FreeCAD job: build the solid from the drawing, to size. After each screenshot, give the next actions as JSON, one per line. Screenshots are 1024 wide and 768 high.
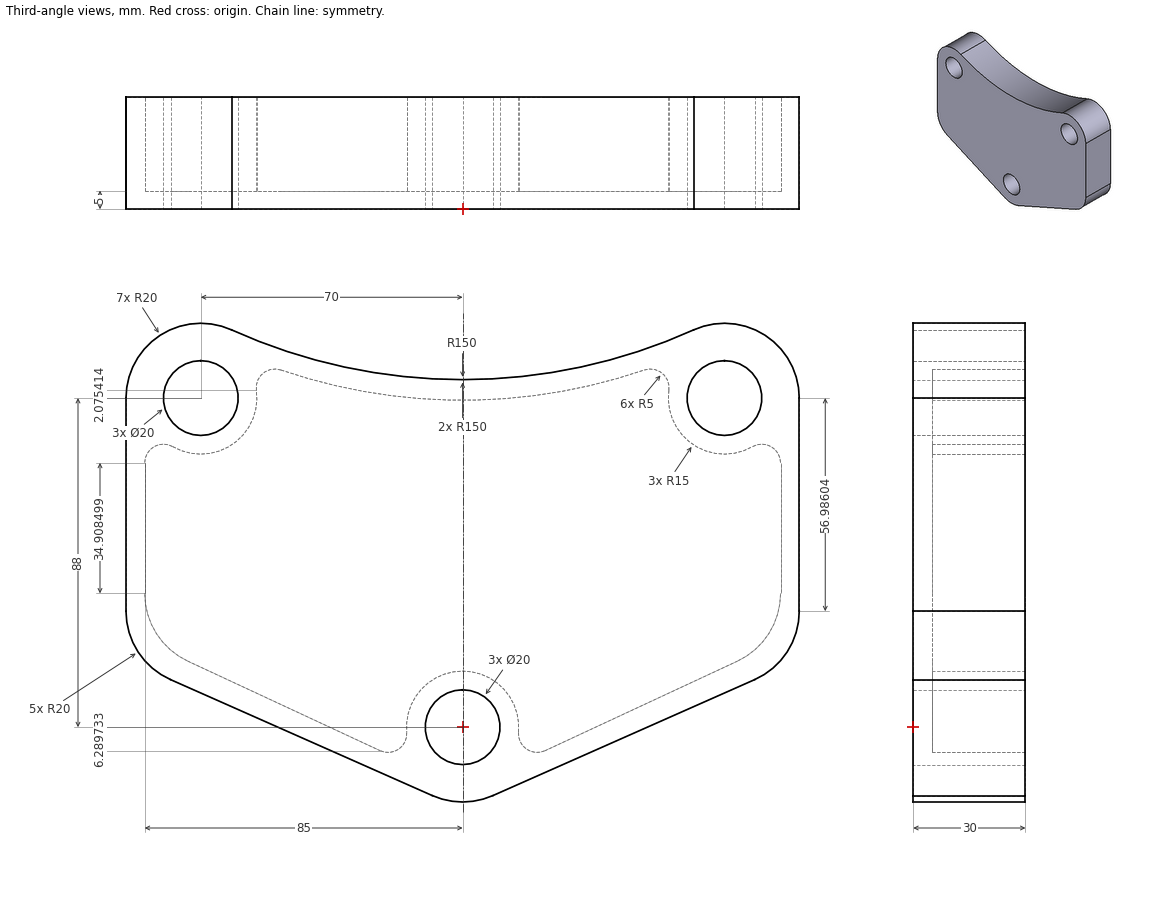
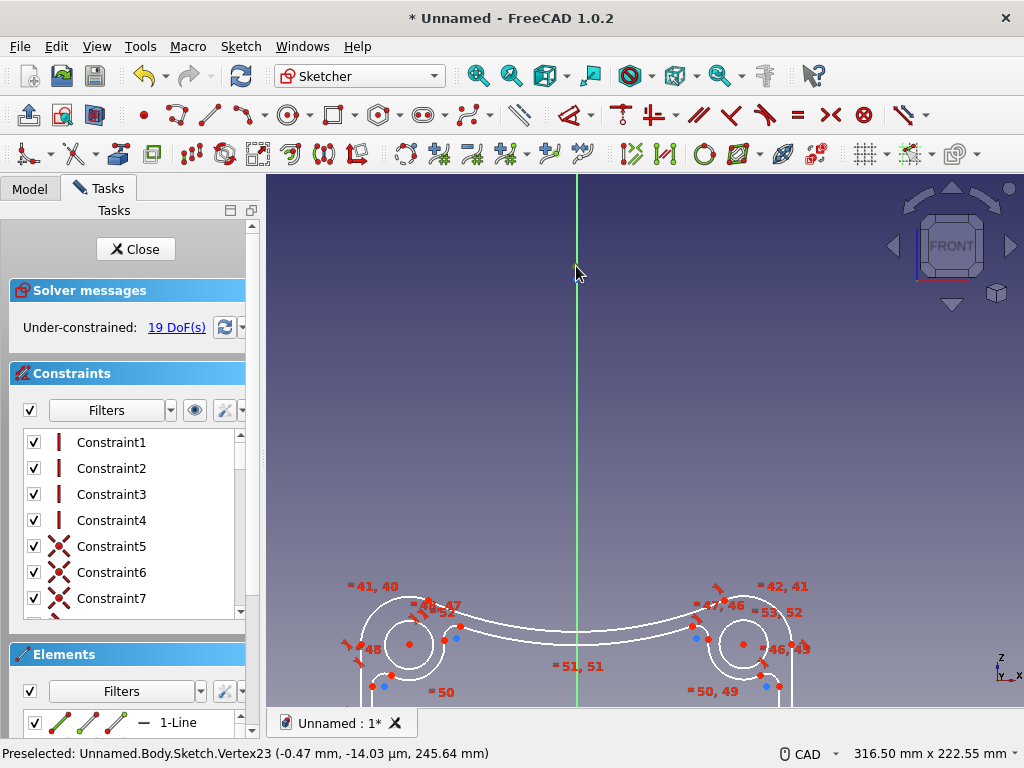
{"action": "left_click", "coordinate": [577, 577]}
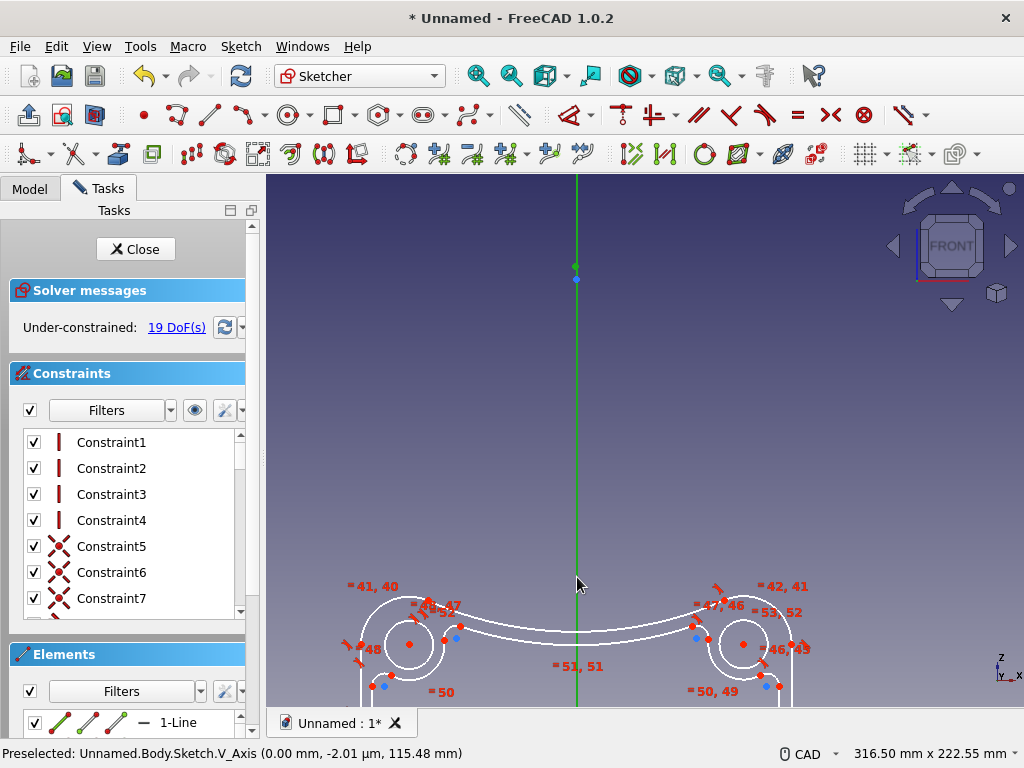
{"action": "left_click", "coordinate": [621, 116]}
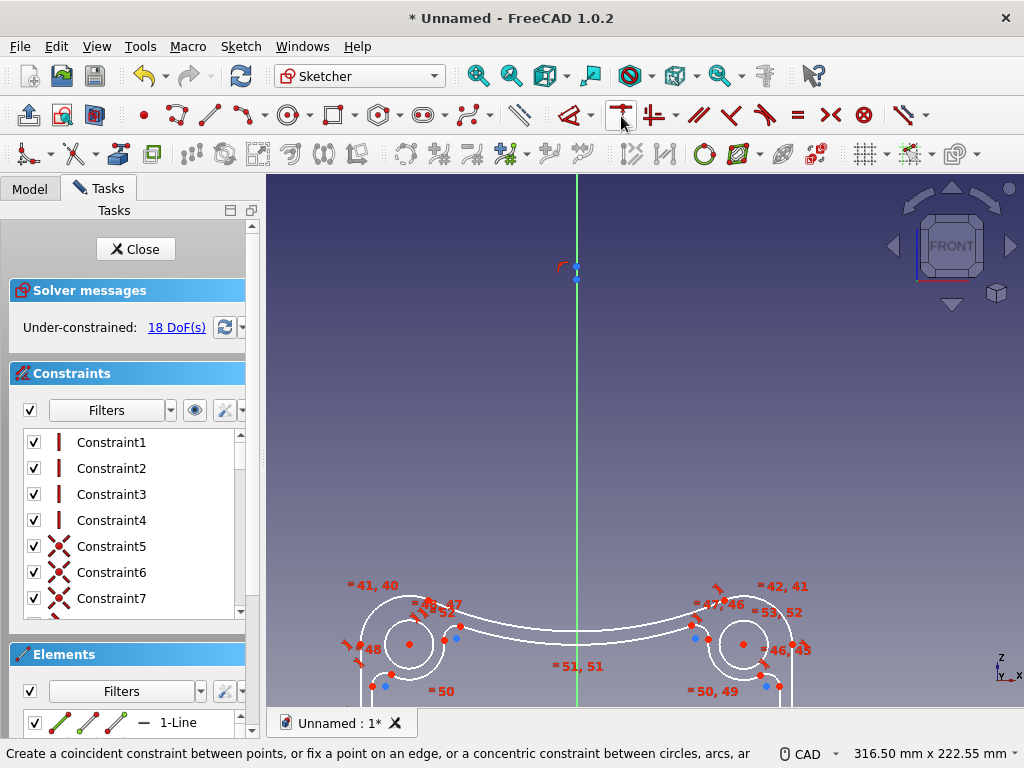
{"action": "left_click", "coordinate": [576, 280]}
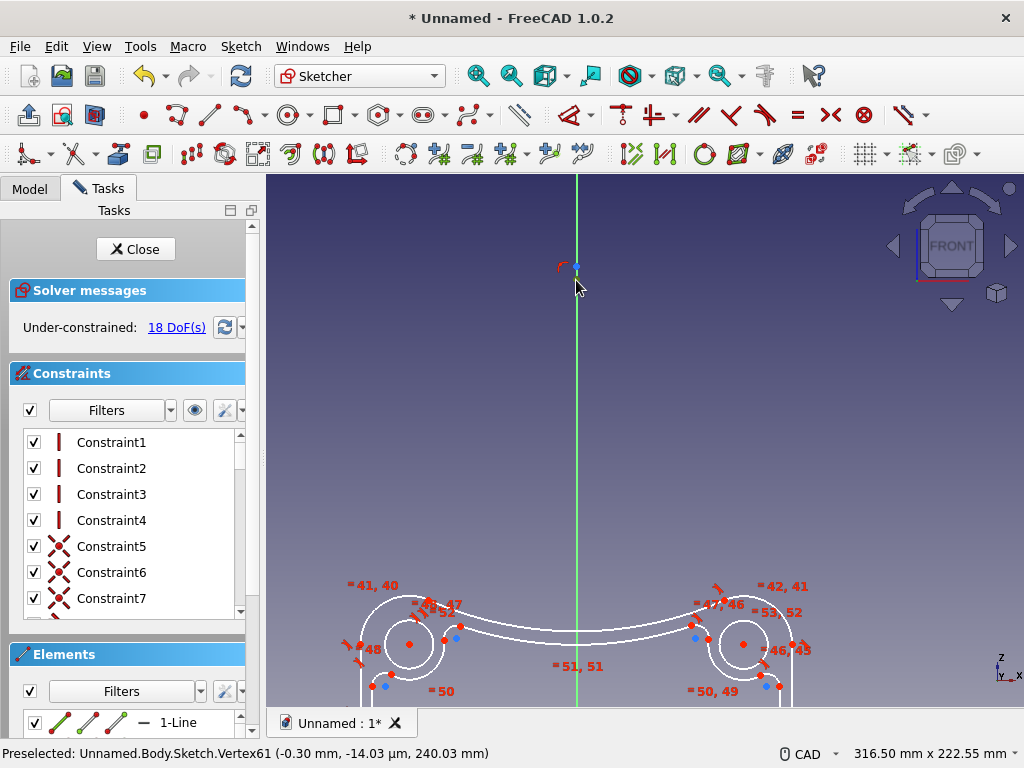
{"action": "left_click", "coordinate": [577, 577]}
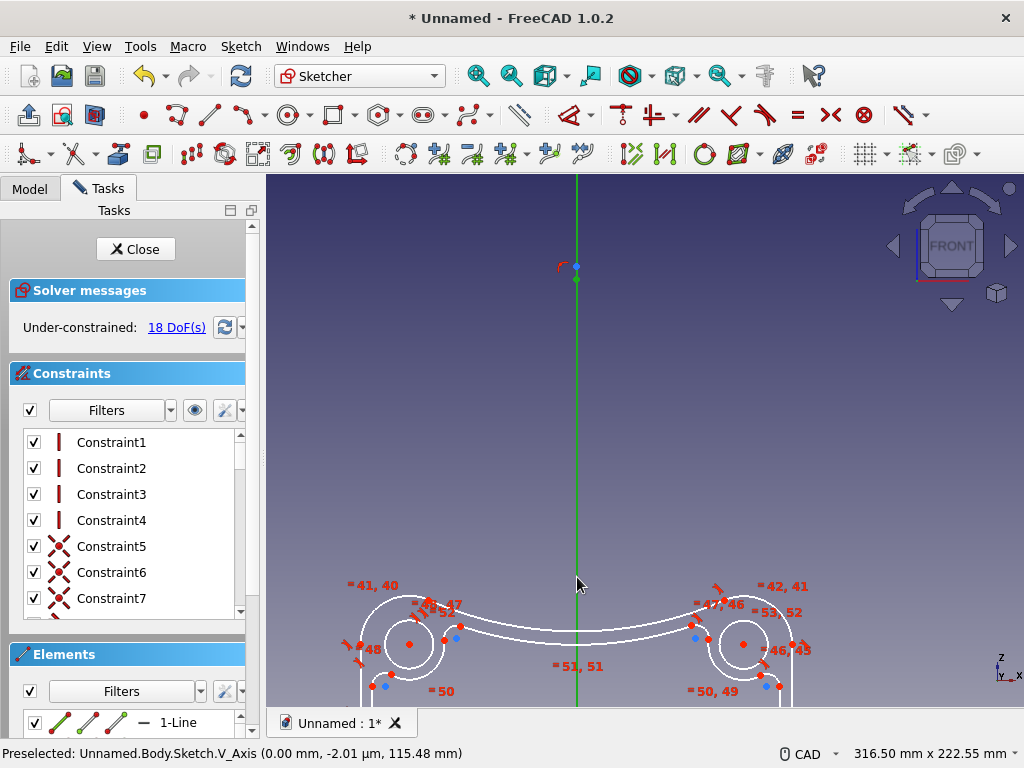
{"action": "left_click", "coordinate": [621, 116]}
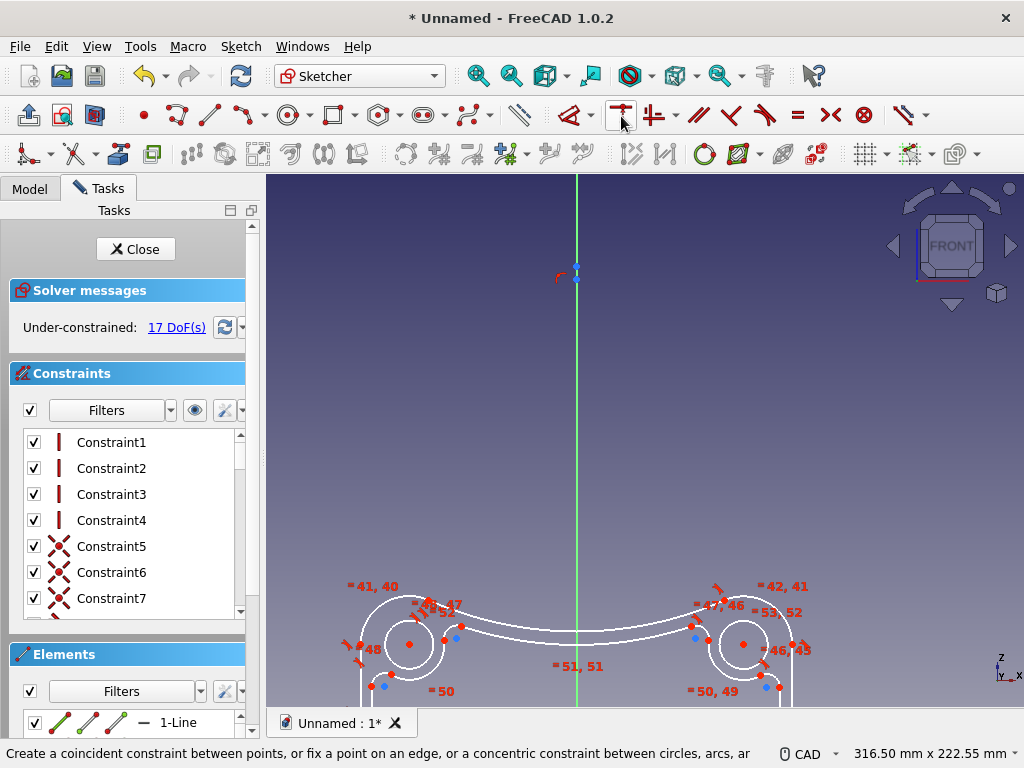
{"action": "scroll", "coordinate": [576, 202], "scroll_direction": "down", "scroll_amount": 3}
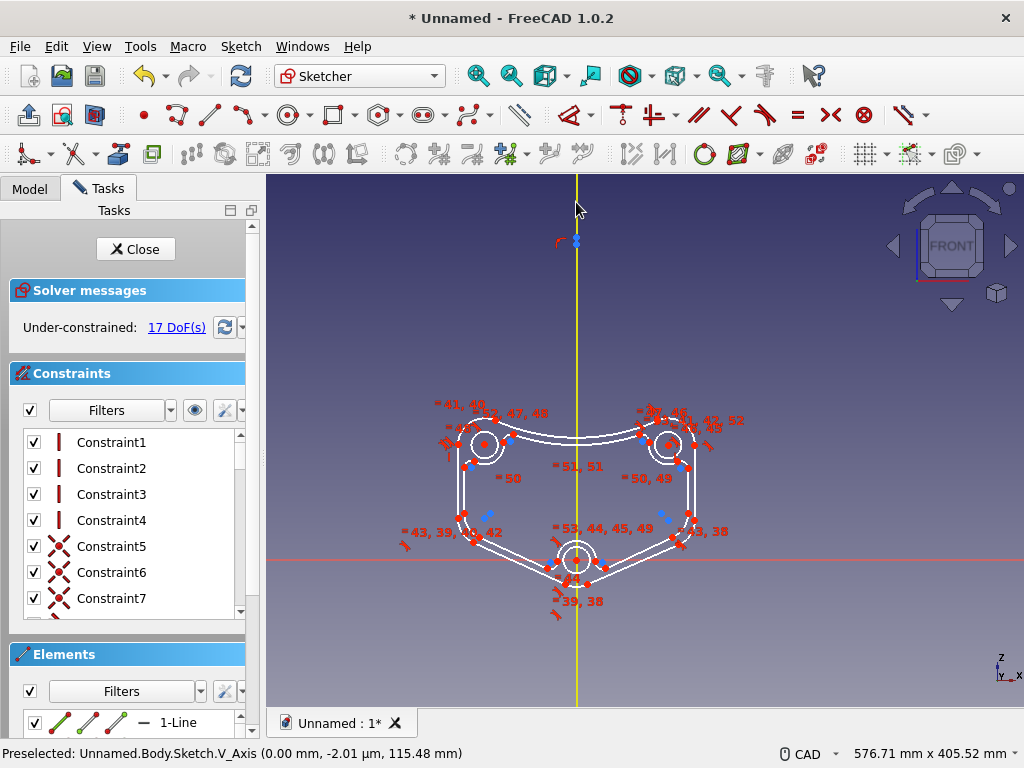
{"action": "scroll", "coordinate": [577, 580], "scroll_direction": "up", "scroll_amount": 3}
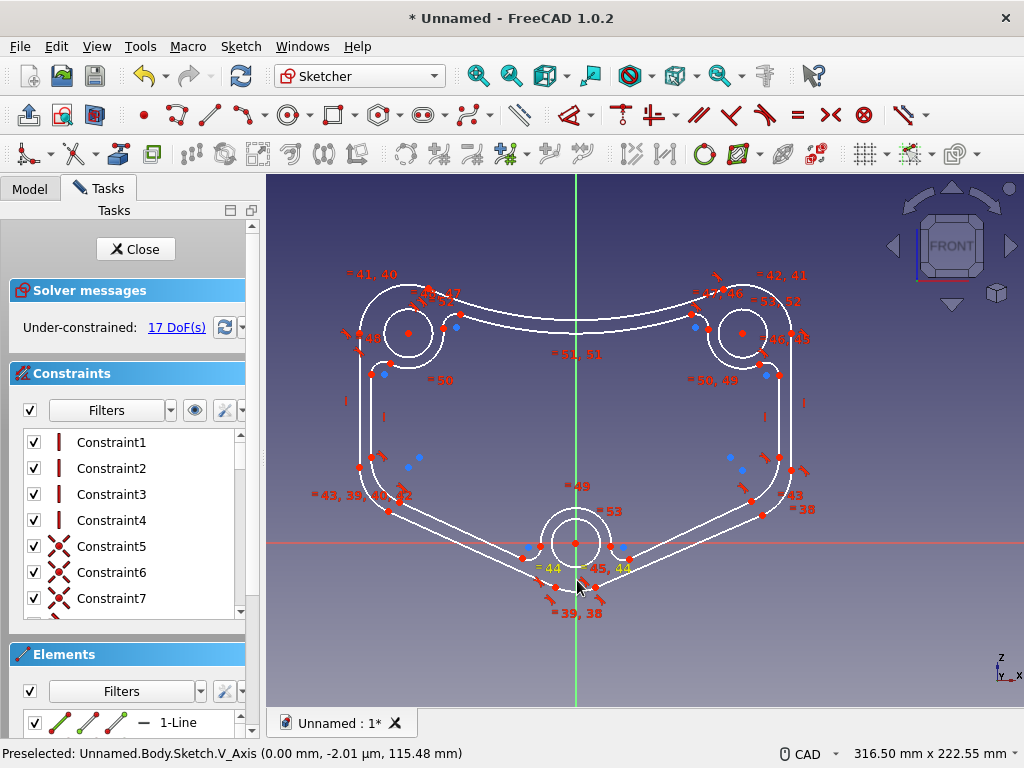
{"action": "left_click", "coordinate": [743, 471]}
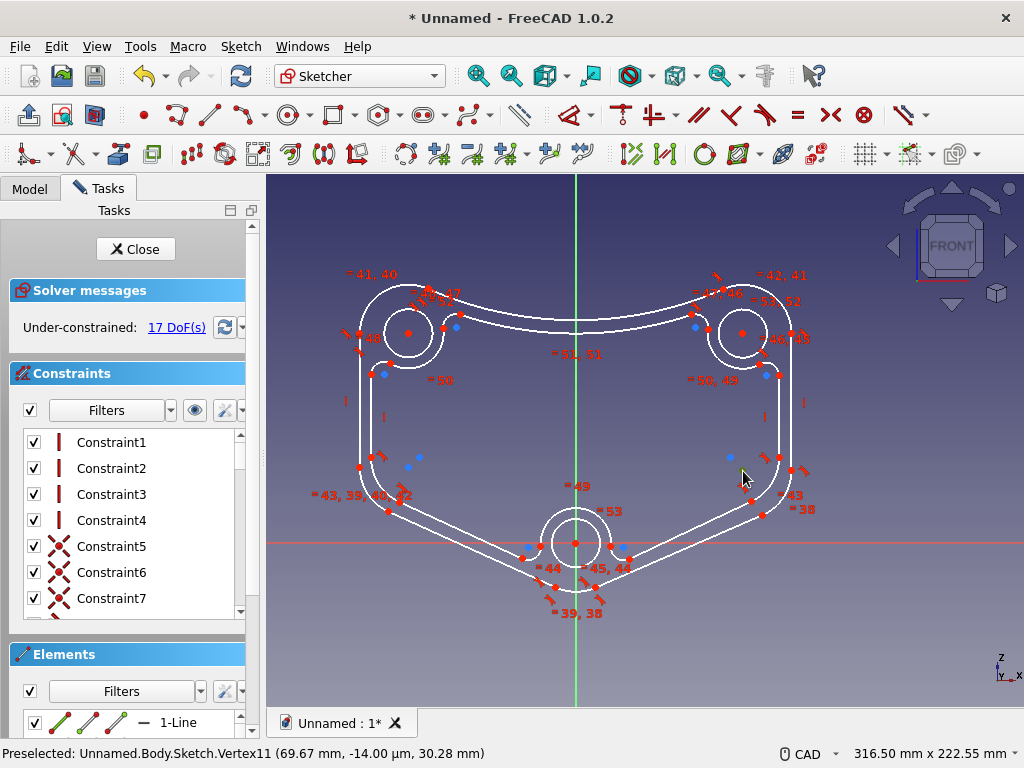
{"action": "left_click", "coordinate": [408, 467]}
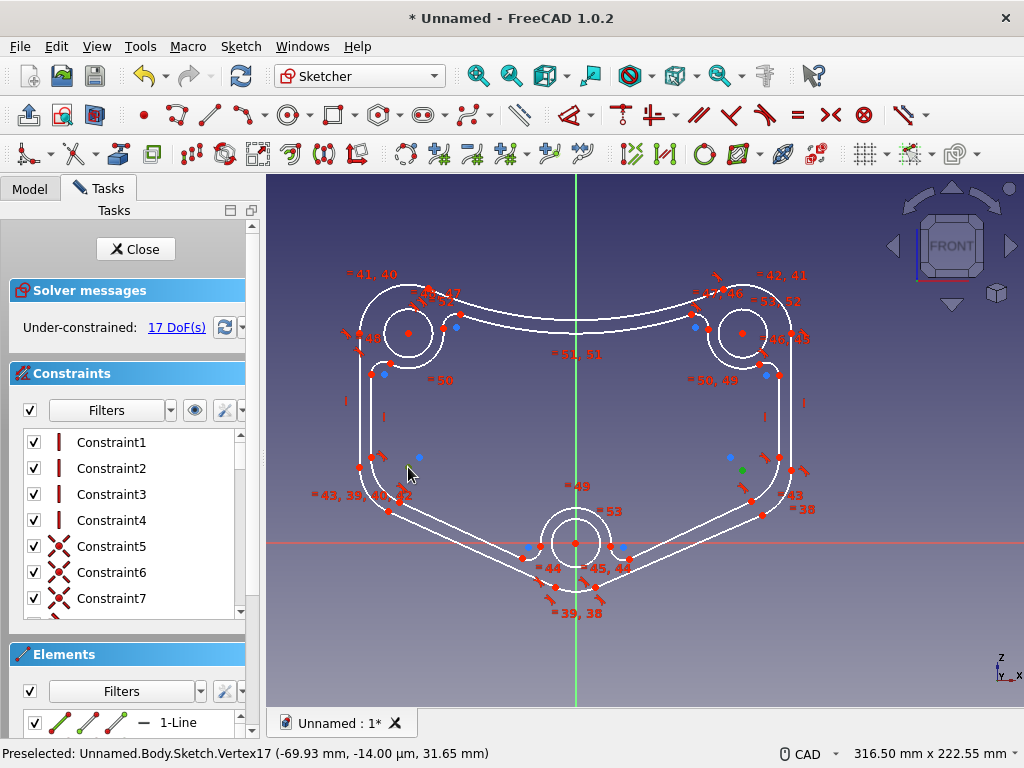
{"action": "left_click", "coordinate": [576, 645]}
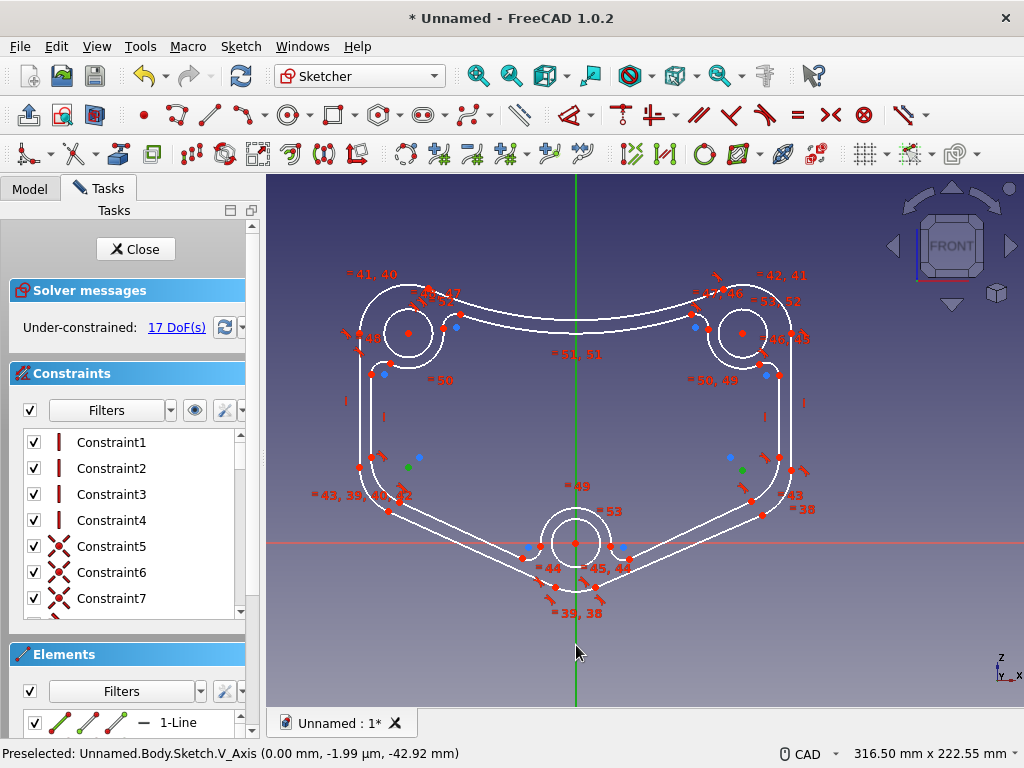
{"action": "left_click", "coordinate": [831, 116]}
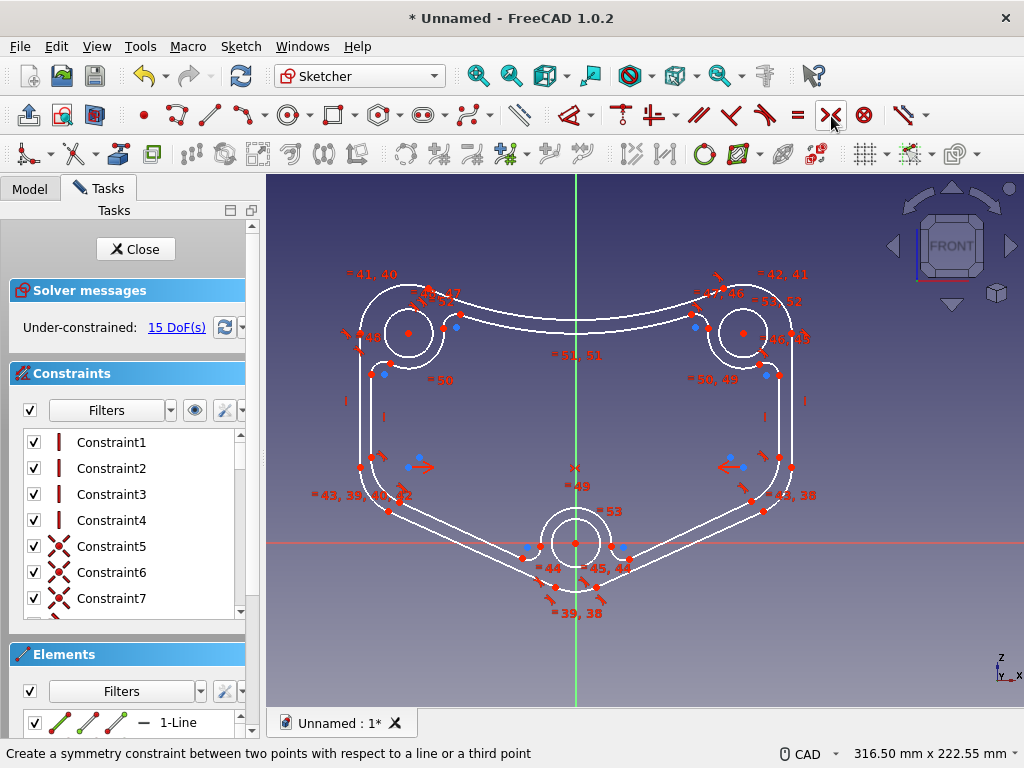
{"action": "left_click", "coordinate": [420, 458]}